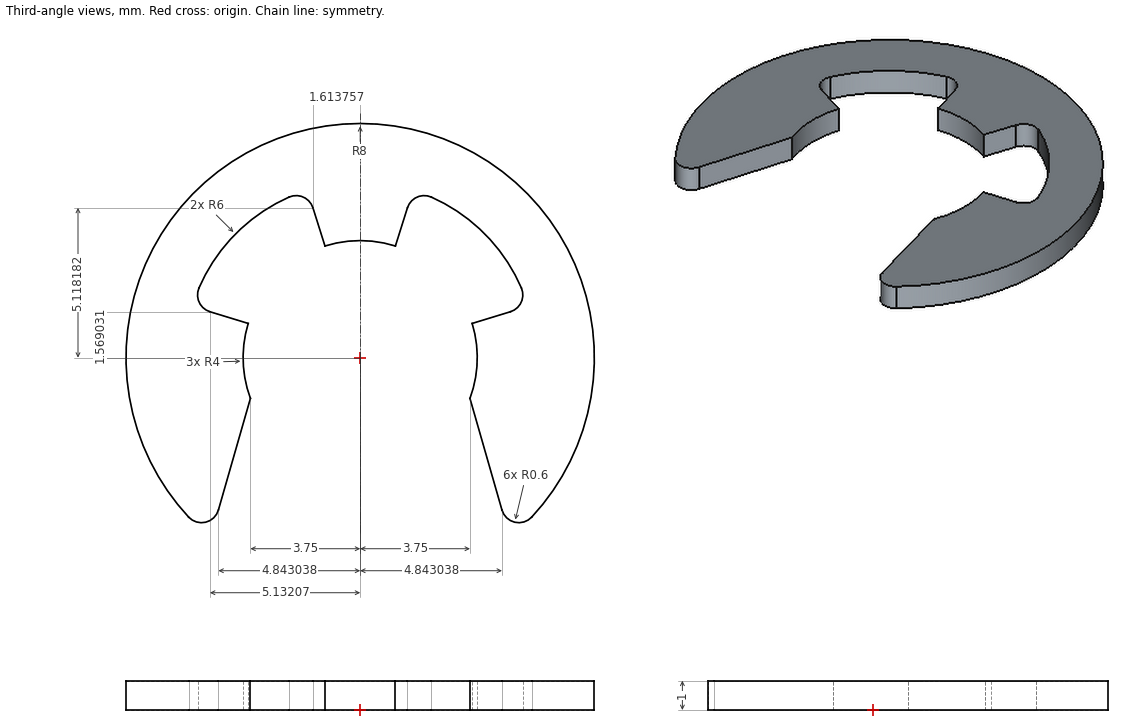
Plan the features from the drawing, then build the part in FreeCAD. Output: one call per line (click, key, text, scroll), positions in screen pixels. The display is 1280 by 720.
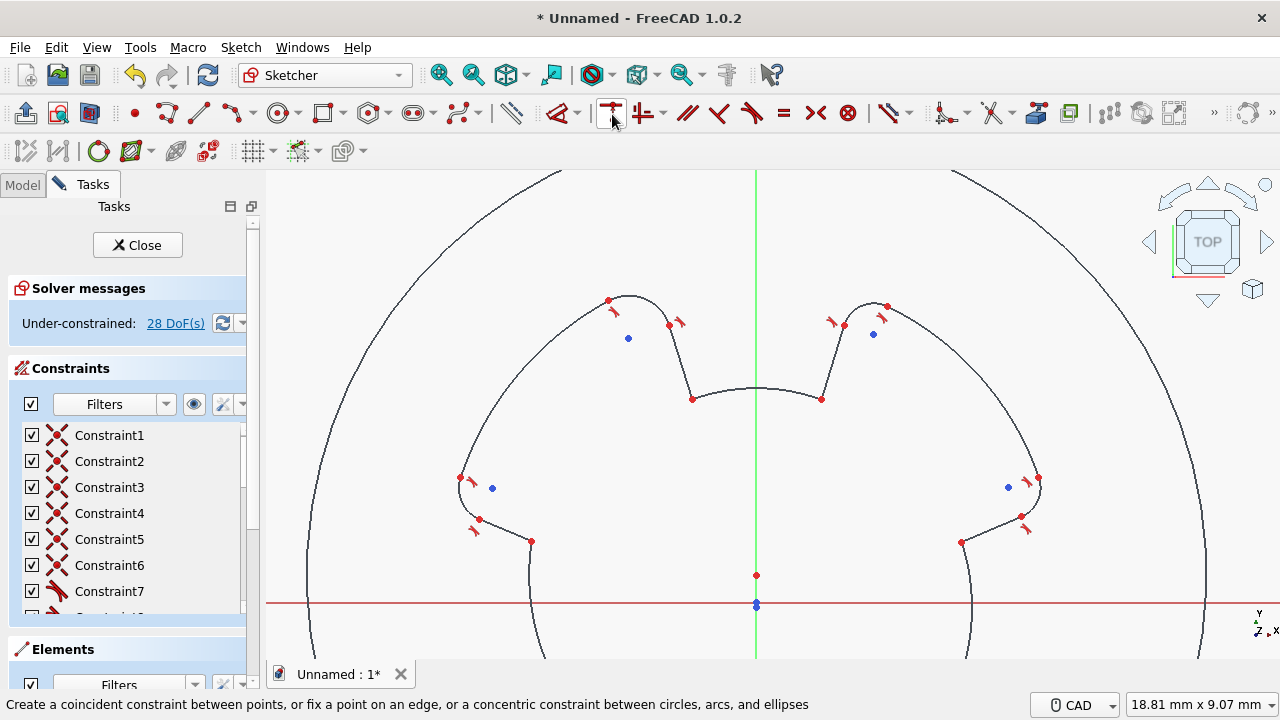
click(391, 312)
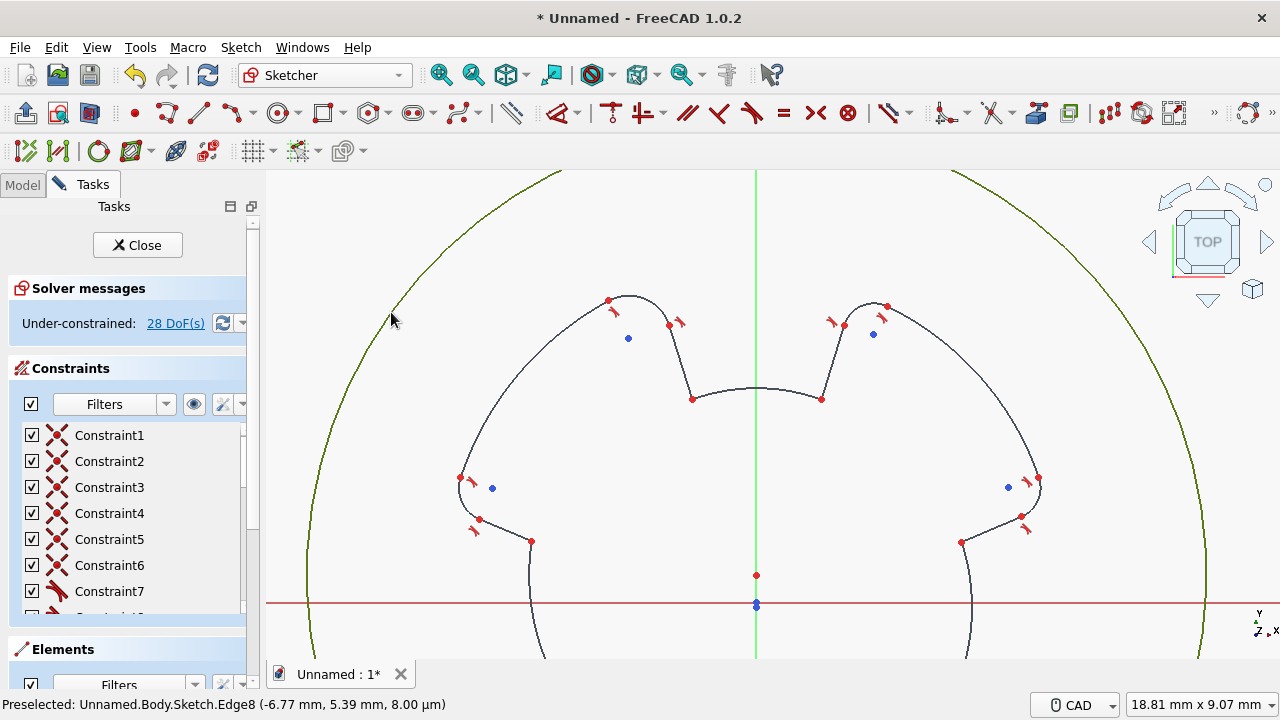
click(971, 583)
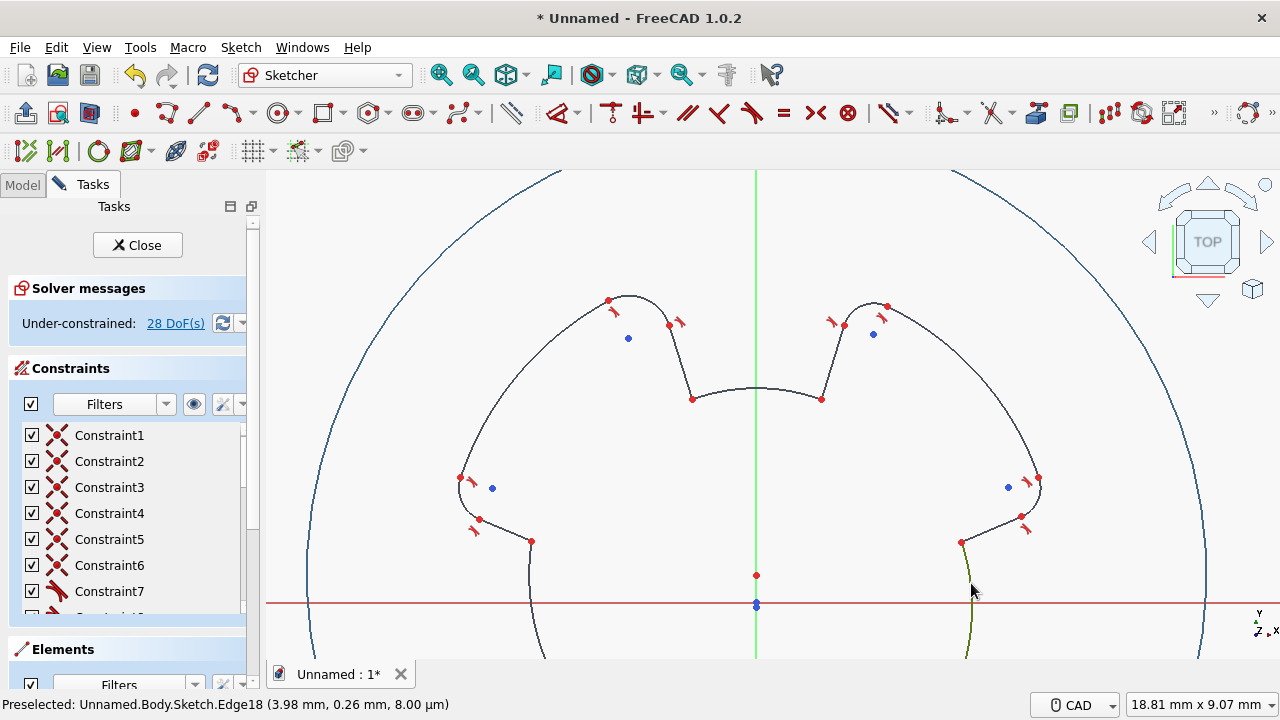
click(612, 114)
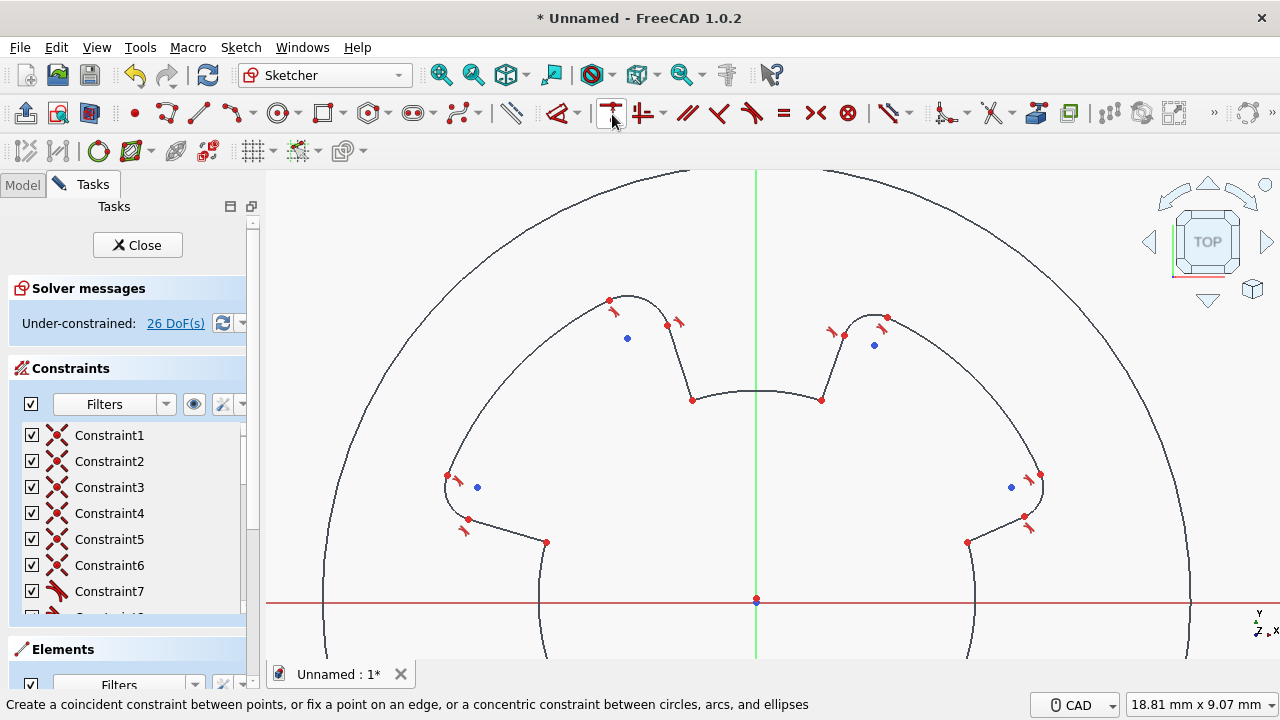
scroll(756, 601, up, 2)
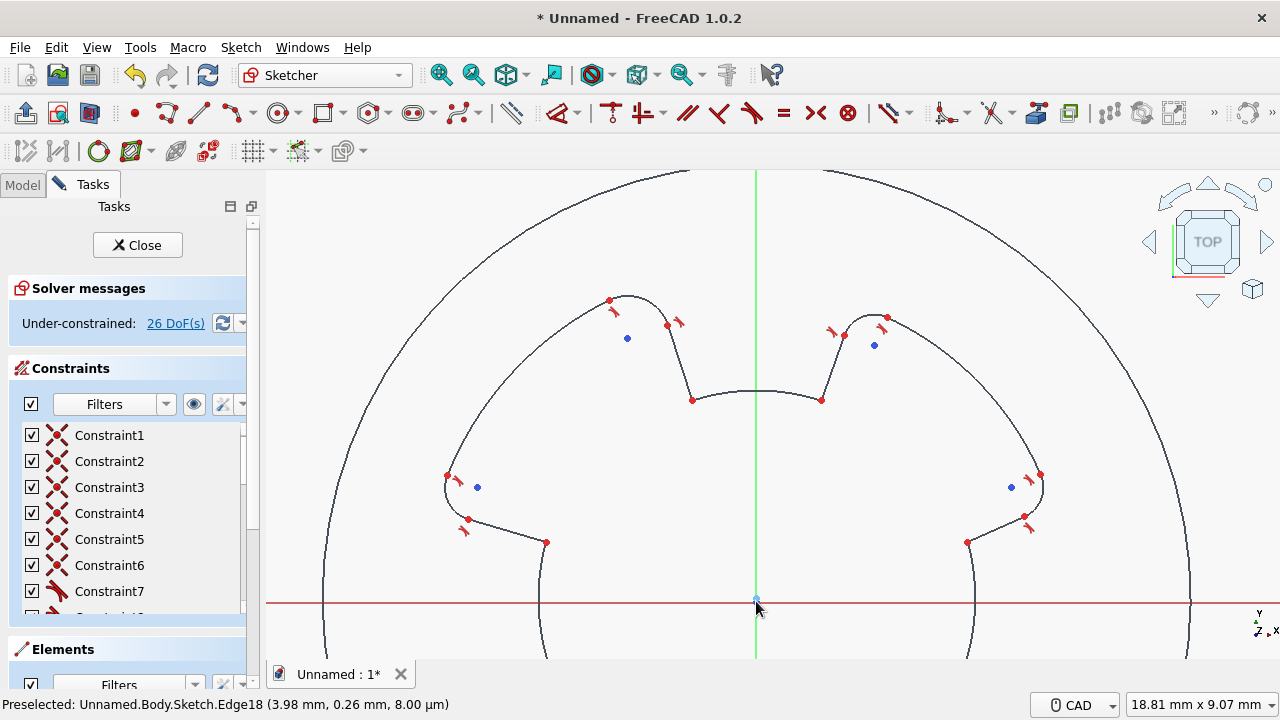
drag(746, 587, 767, 613)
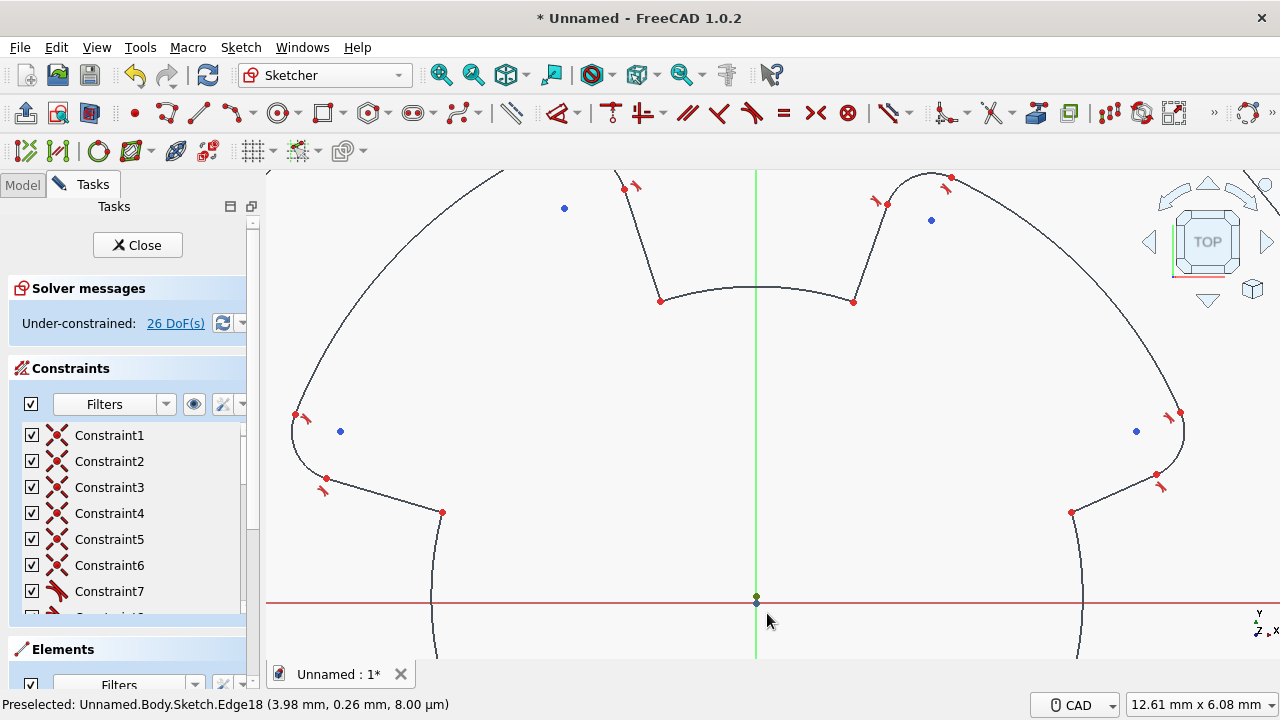
click(612, 114)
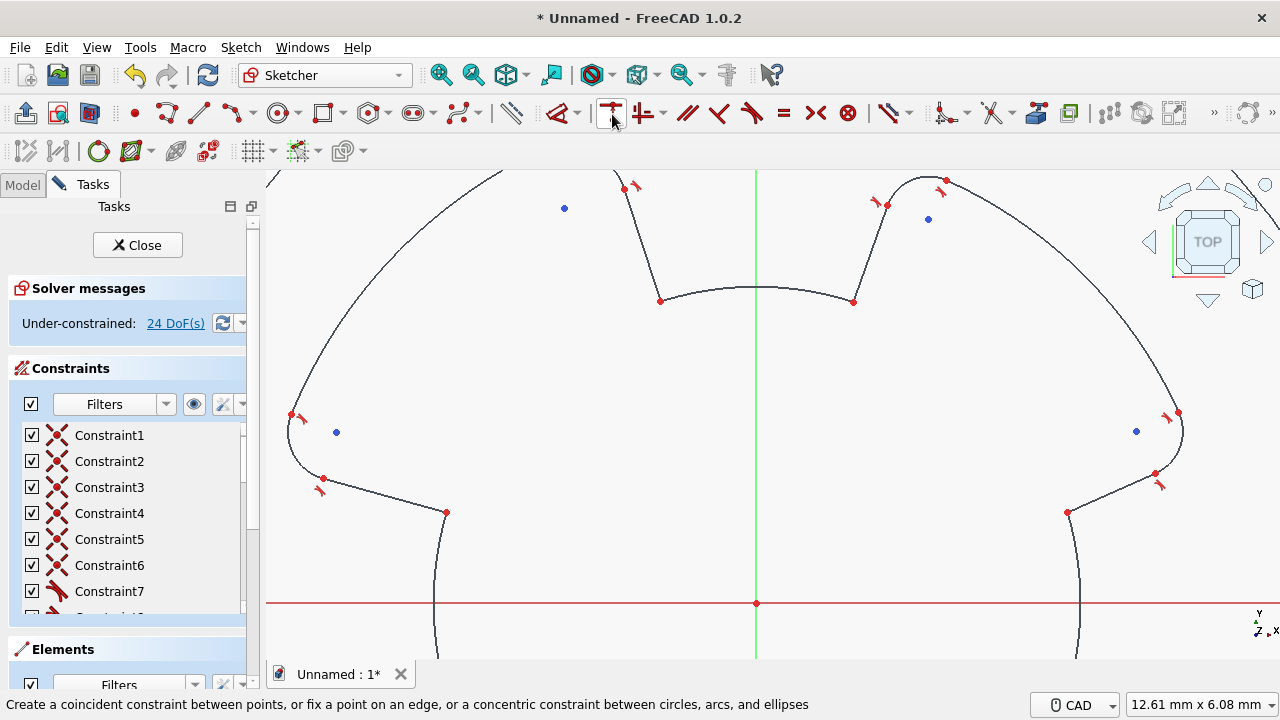
scroll(682, 374, down, 6)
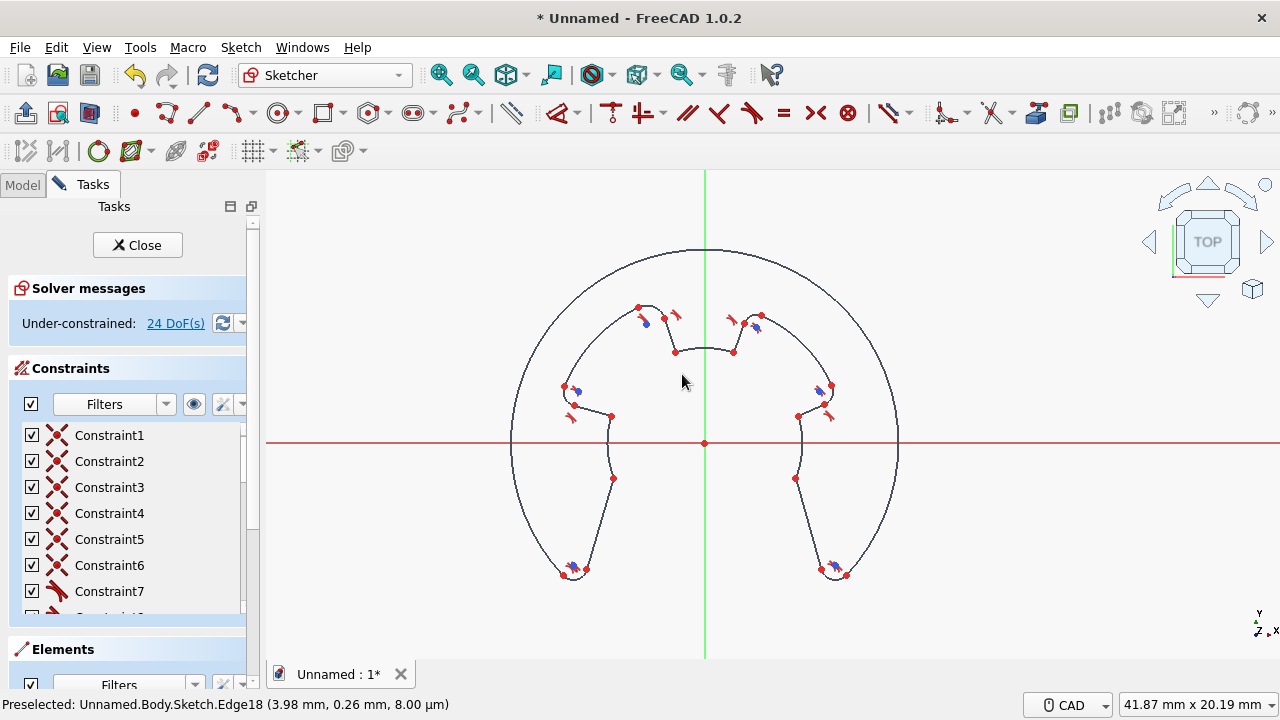
scroll(827, 577, up, 2)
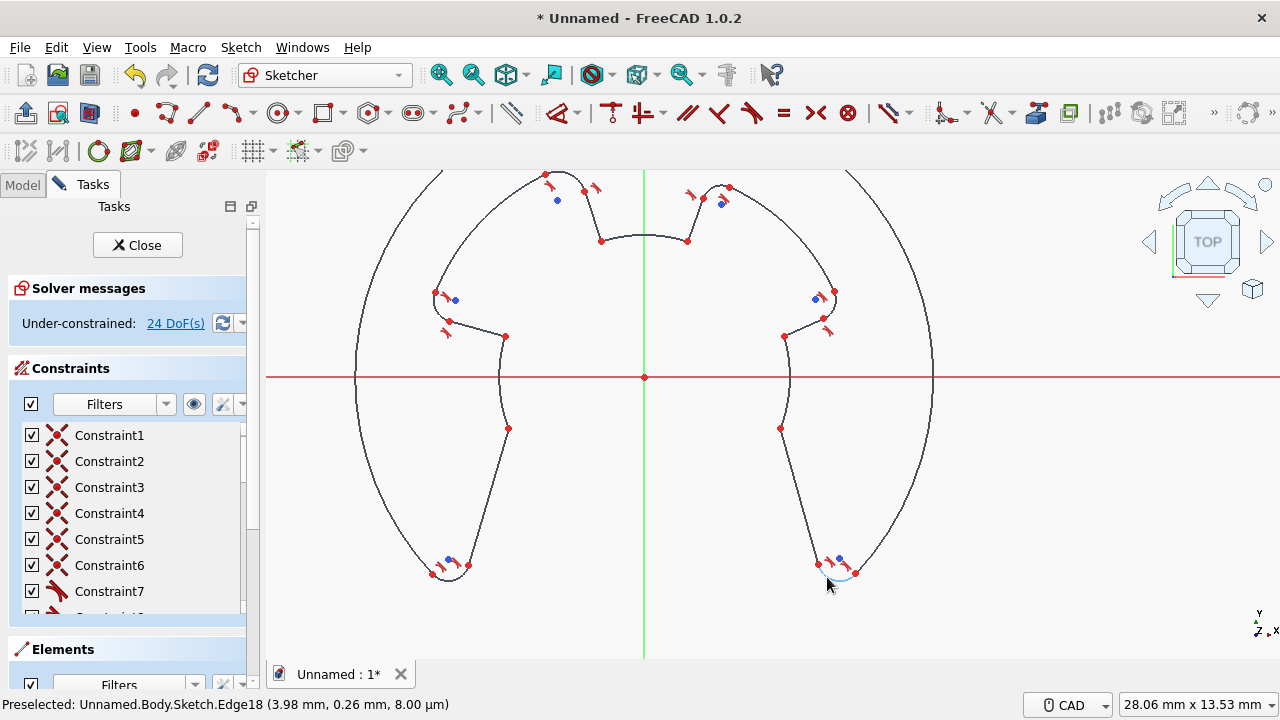
click(826, 576)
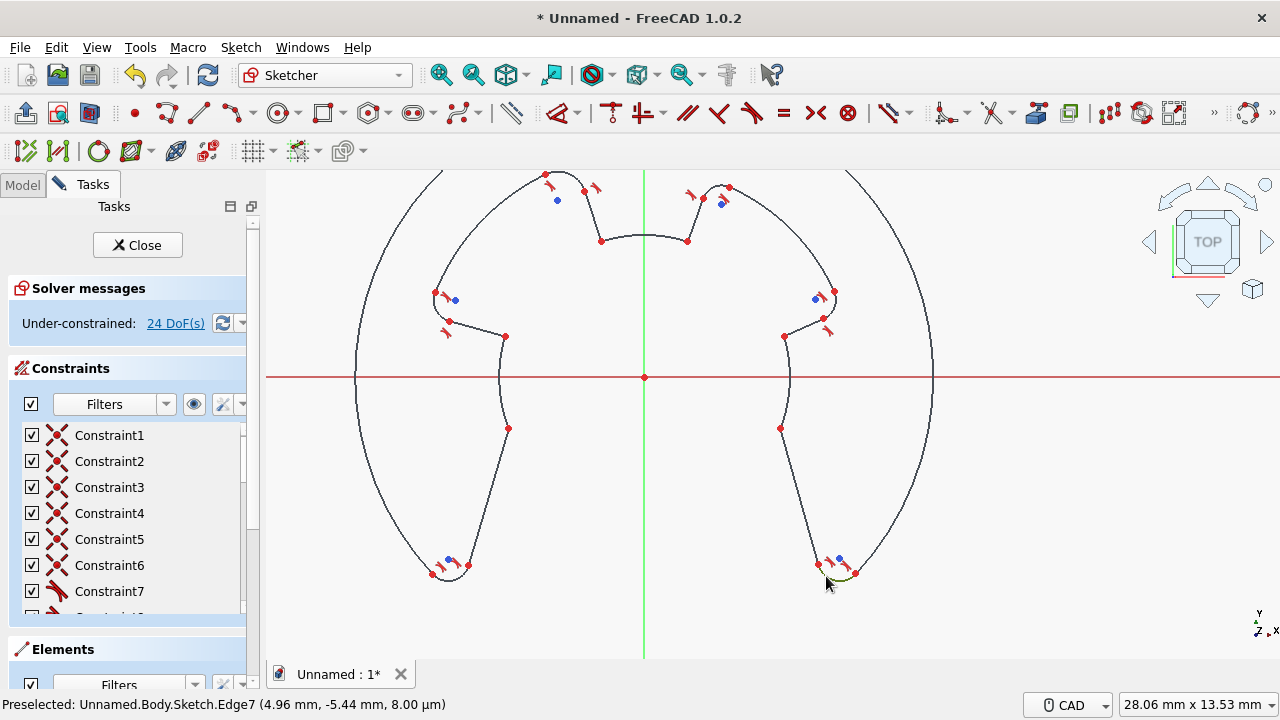
click(444, 581)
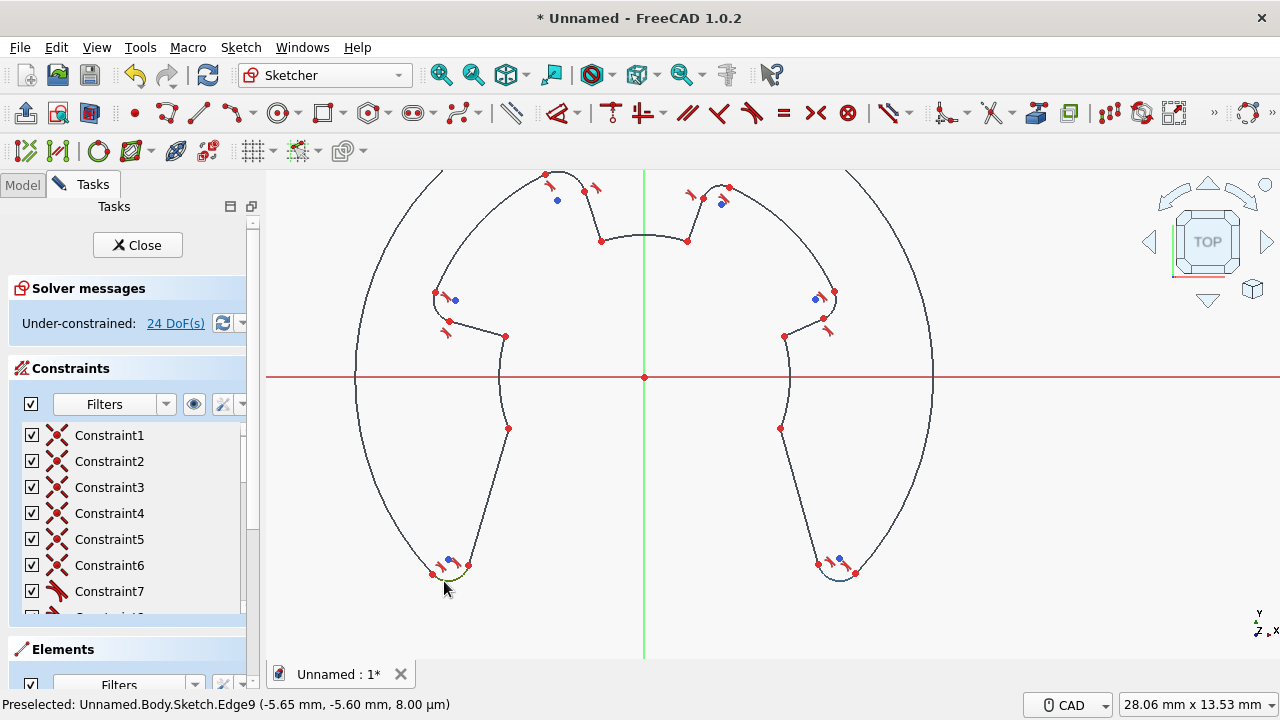
scroll(434, 303, up, 2)